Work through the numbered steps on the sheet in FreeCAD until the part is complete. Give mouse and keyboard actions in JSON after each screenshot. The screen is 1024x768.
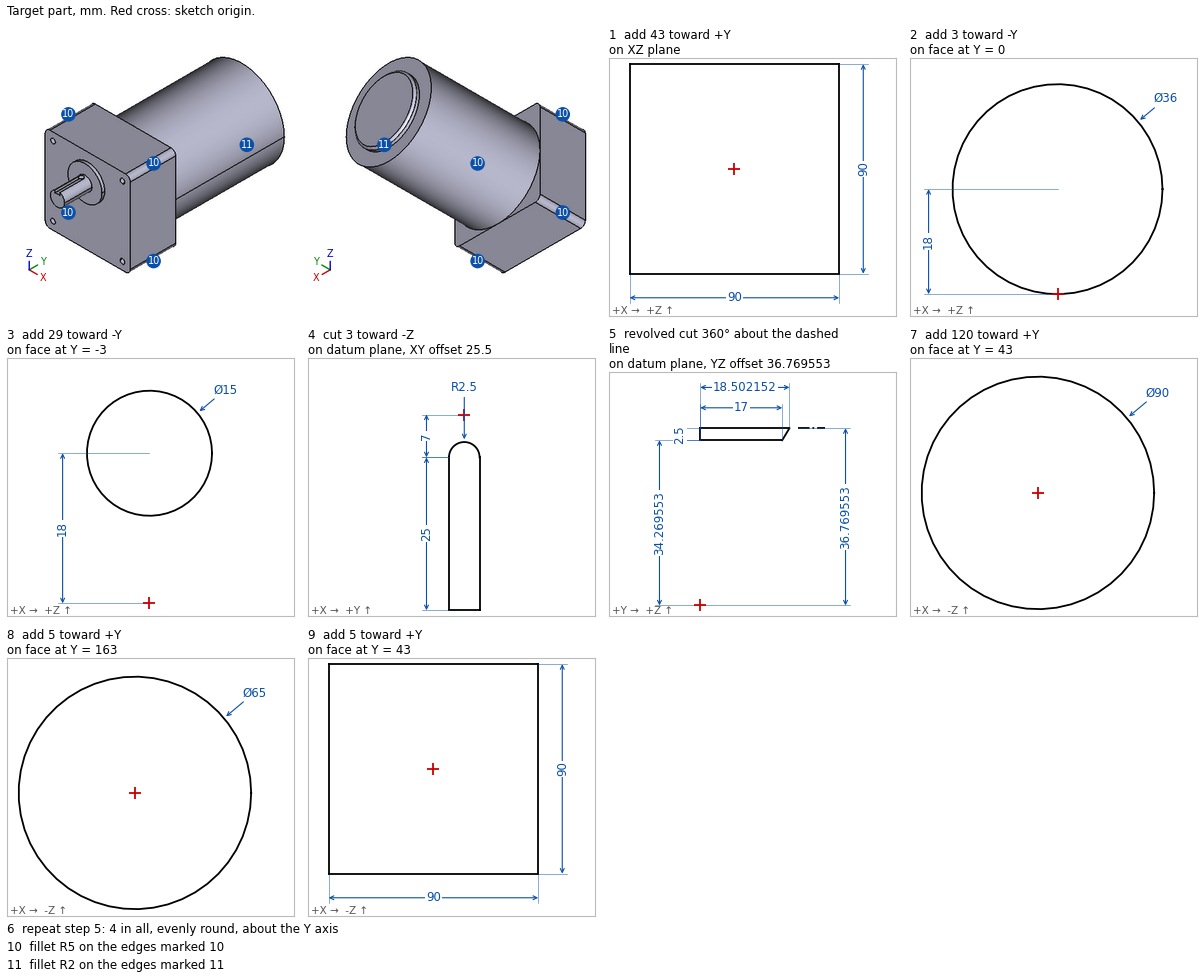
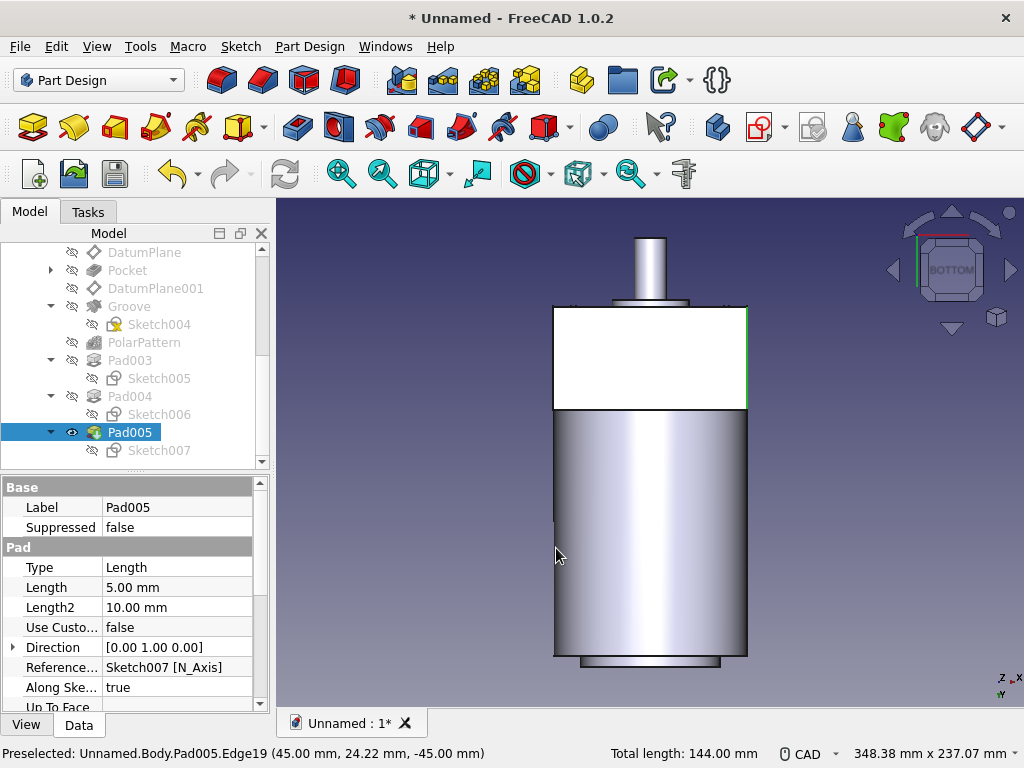
{"action": "left_click", "coordinate": [553, 357], "text": "ctrl"}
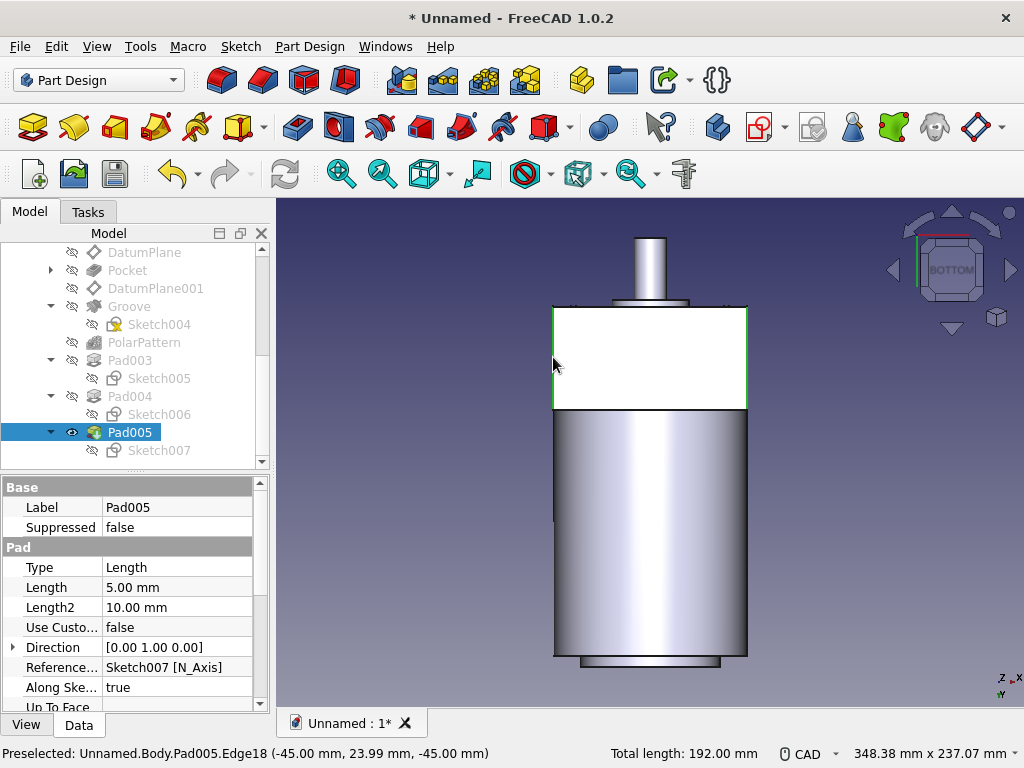
{"action": "left_click", "coordinate": [222, 80]}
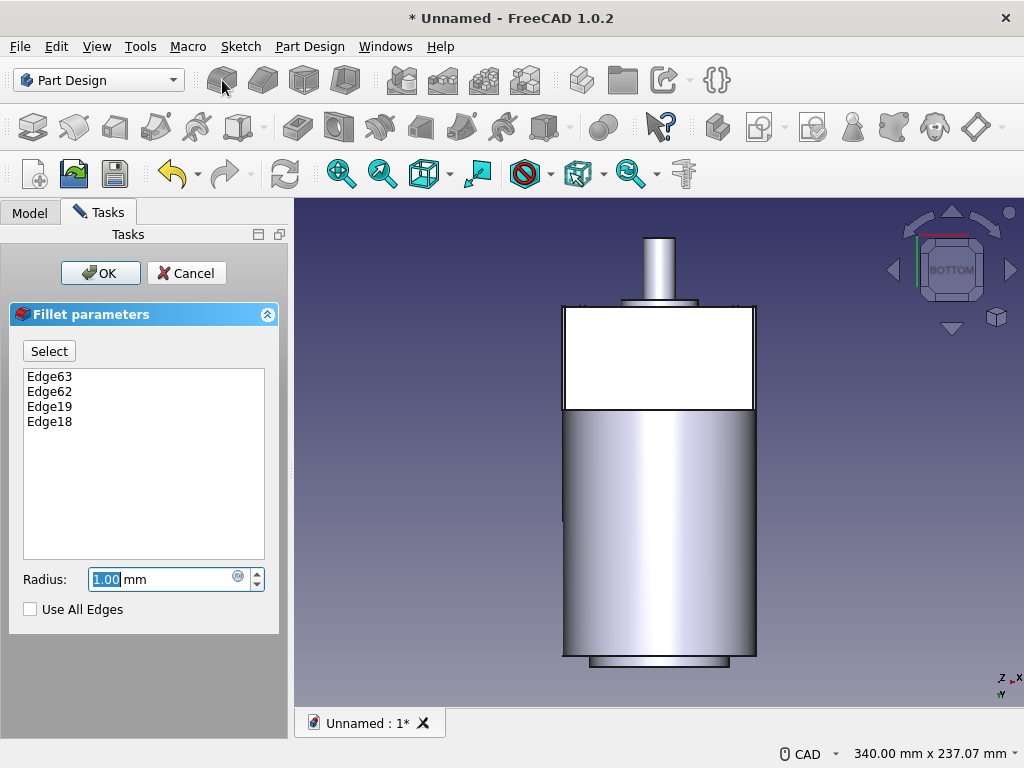
{"action": "type", "text": "5"}
{"action": "key", "text": "Tab"}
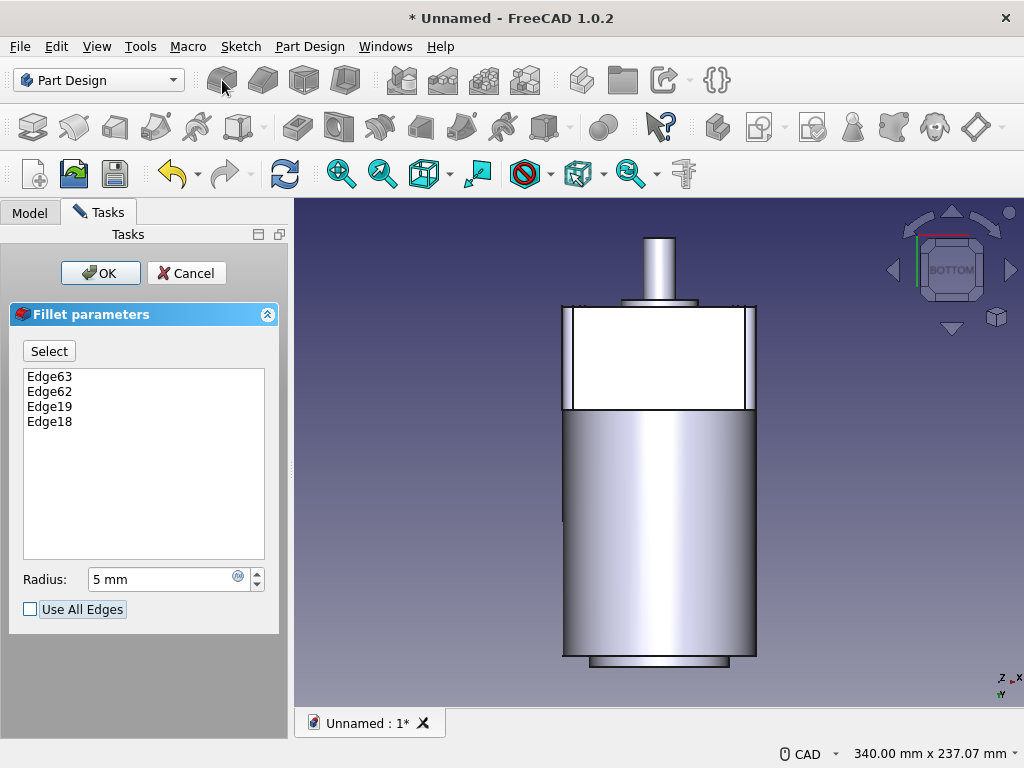
{"action": "left_click", "coordinate": [101, 273]}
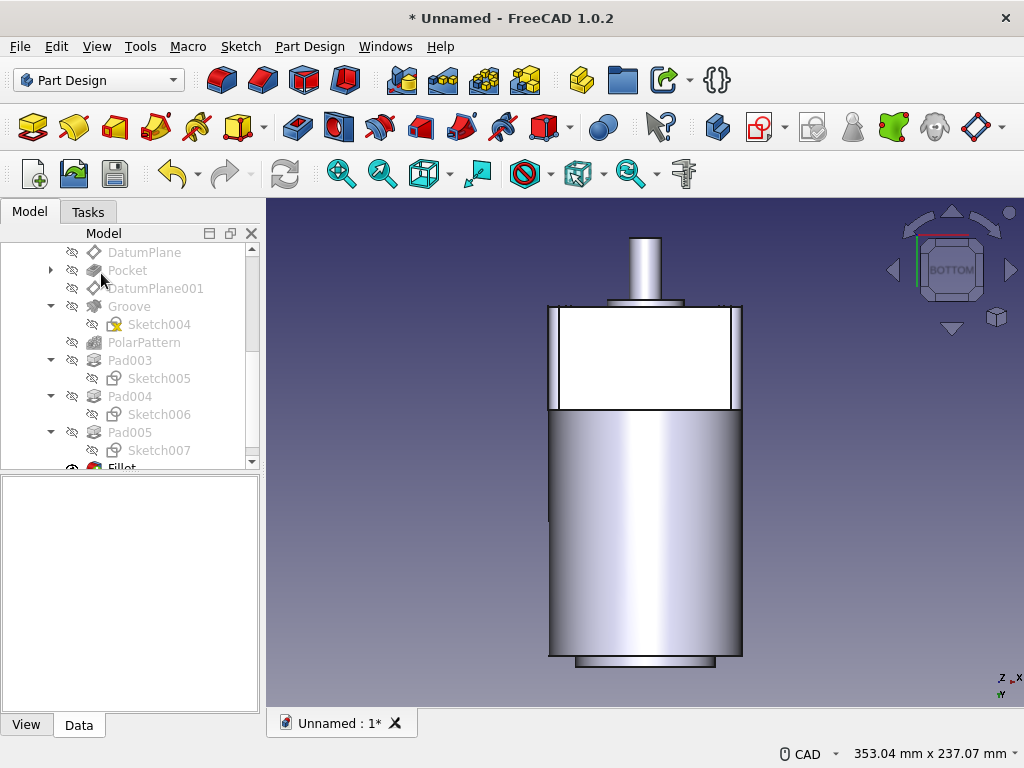
{"action": "key", "text": "0"}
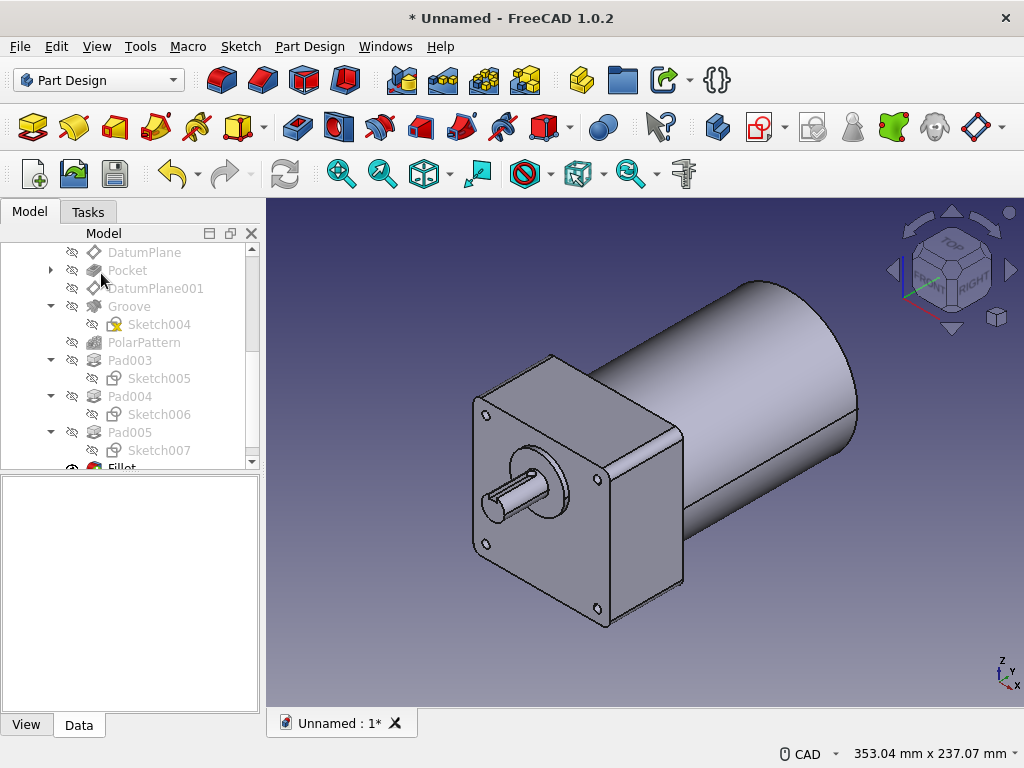
{"action": "key", "text": "2"}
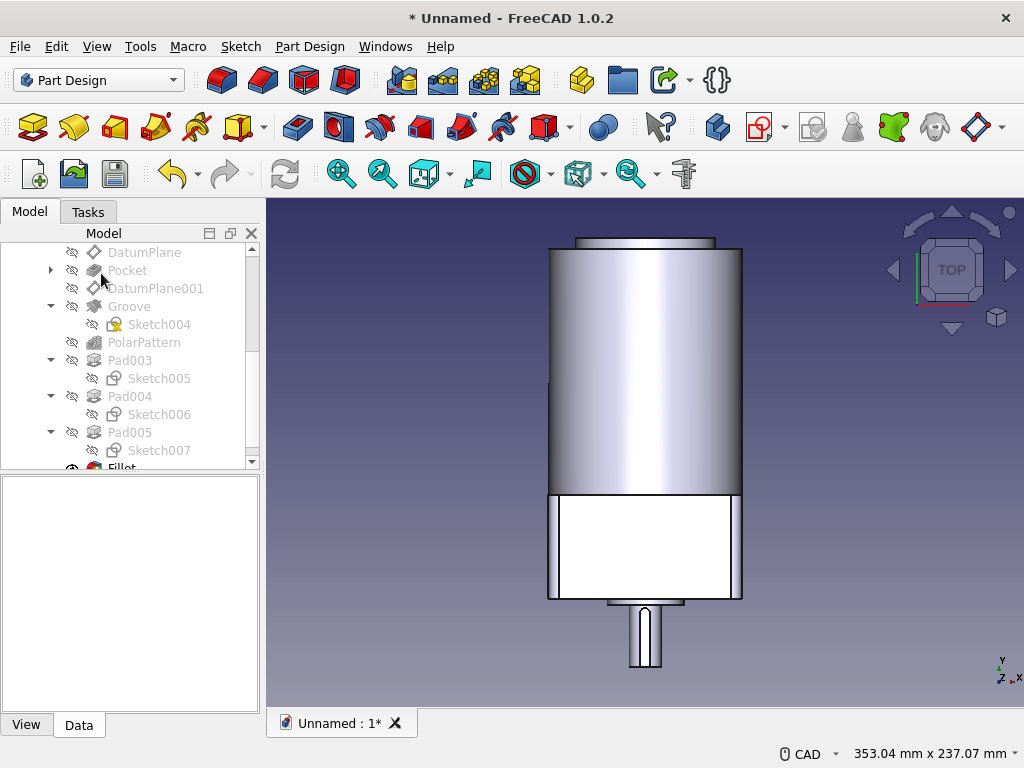
{"action": "left_click", "coordinate": [589, 237]}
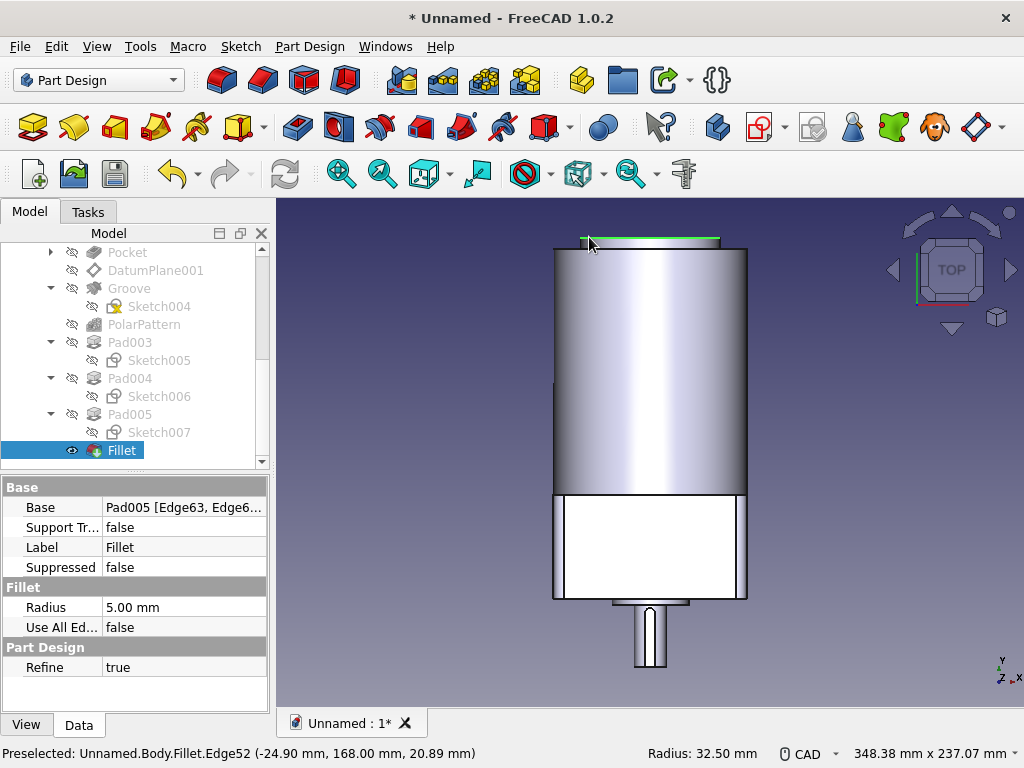
{"action": "left_click", "coordinate": [222, 80]}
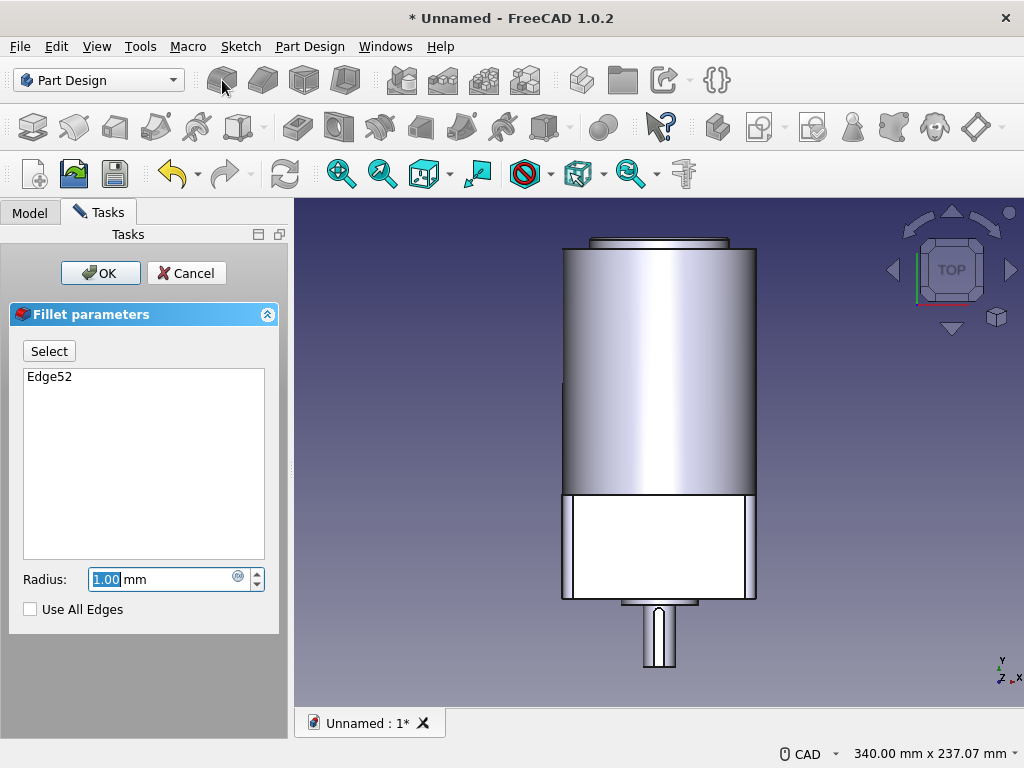
{"action": "type", "text": "2"}
{"action": "key", "text": "Tab"}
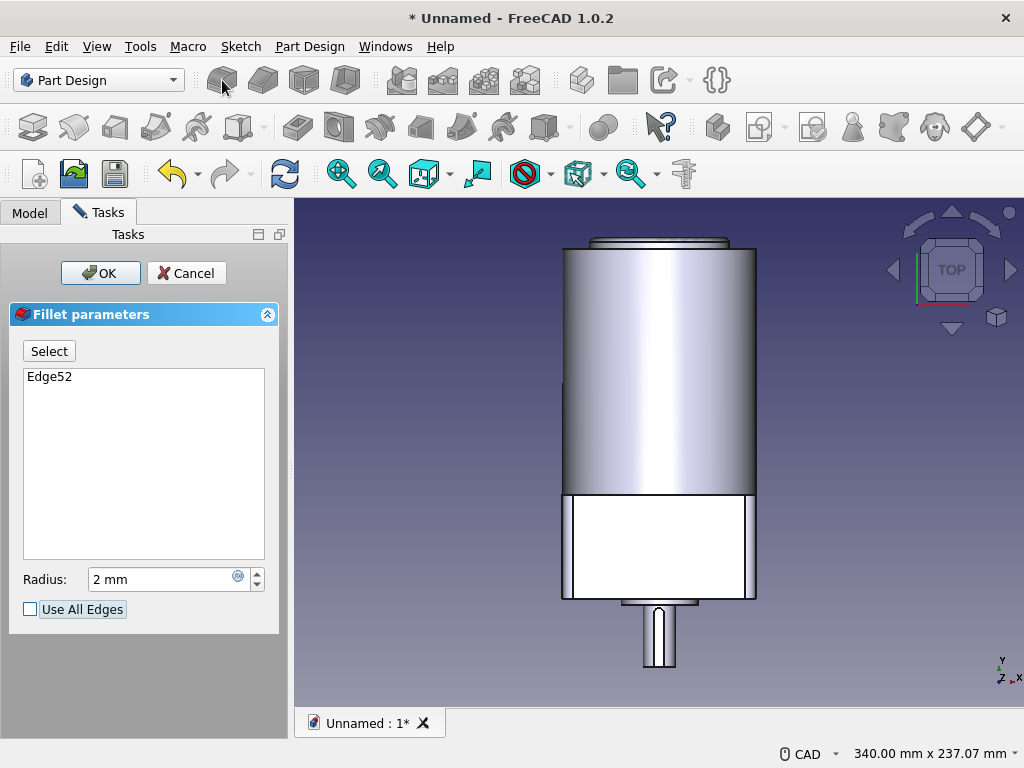
{"action": "left_click", "coordinate": [101, 273]}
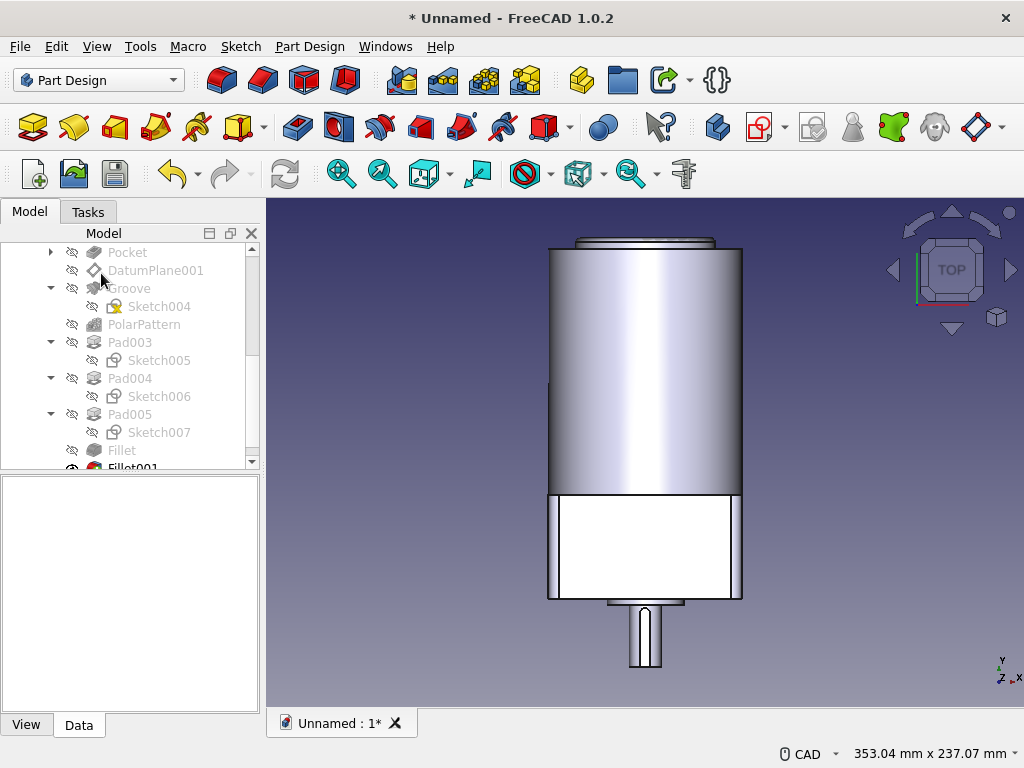
{"action": "key", "text": "0"}